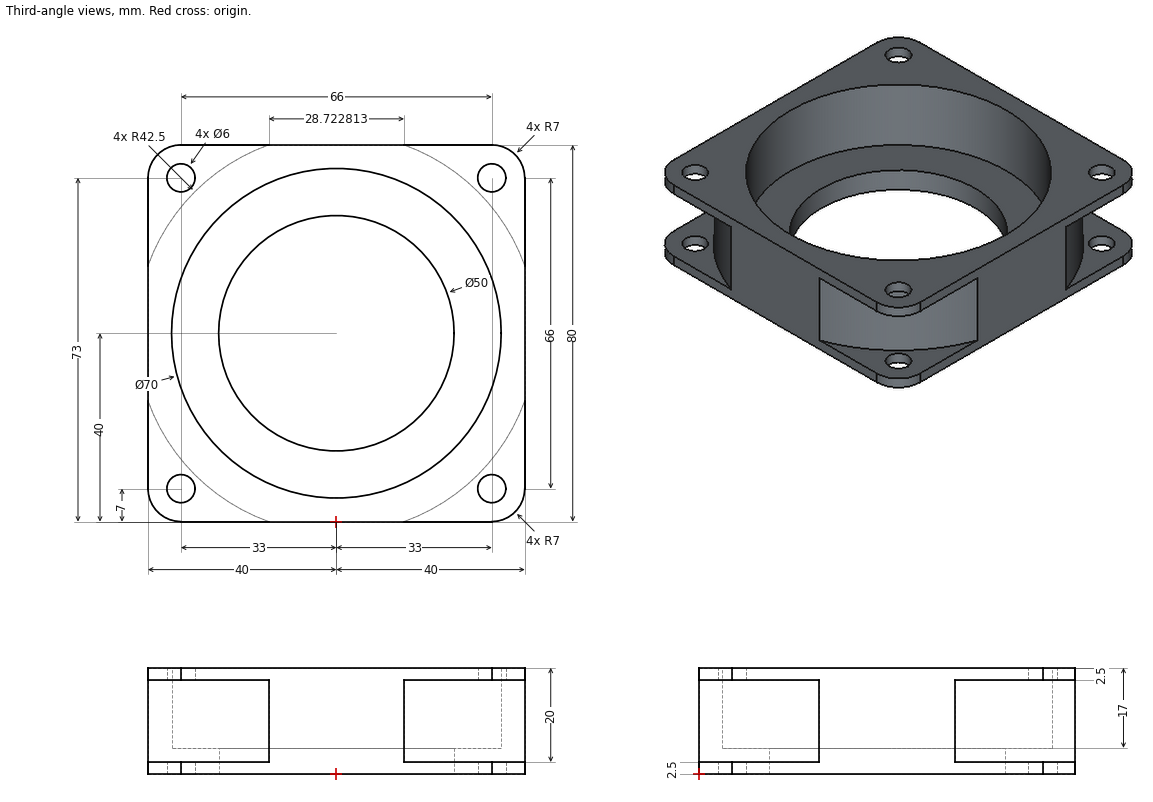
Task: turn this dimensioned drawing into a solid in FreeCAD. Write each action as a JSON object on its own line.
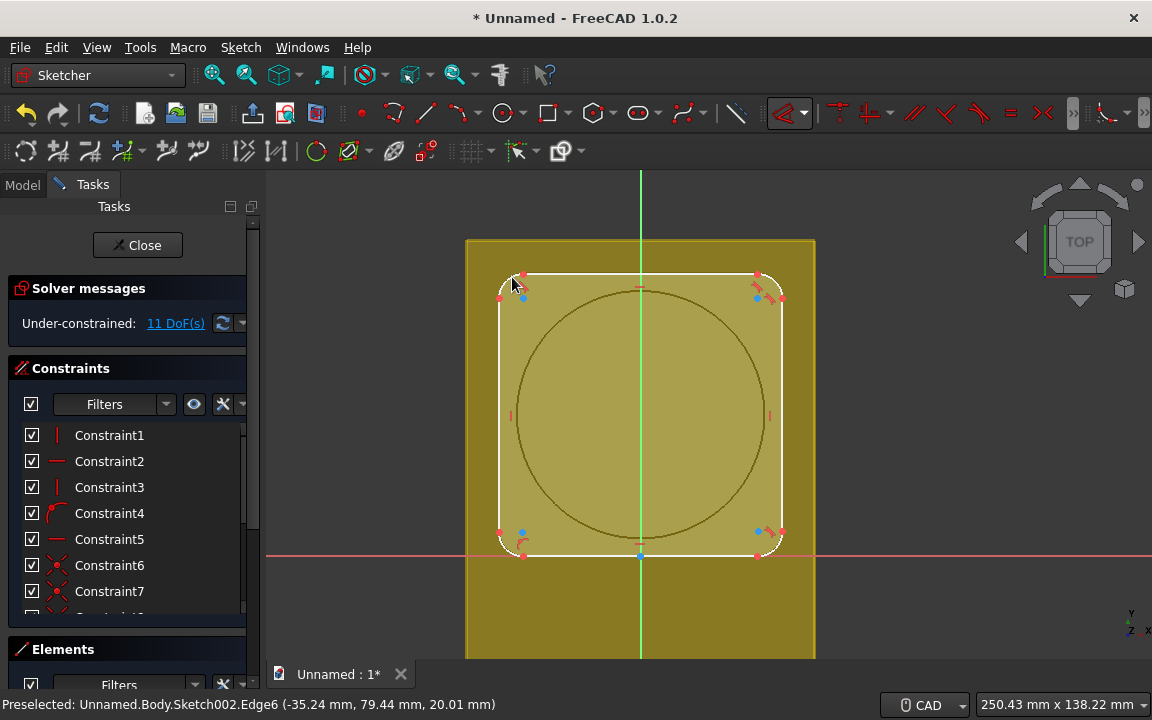
{"action": "left_click", "coordinate": [499, 369]}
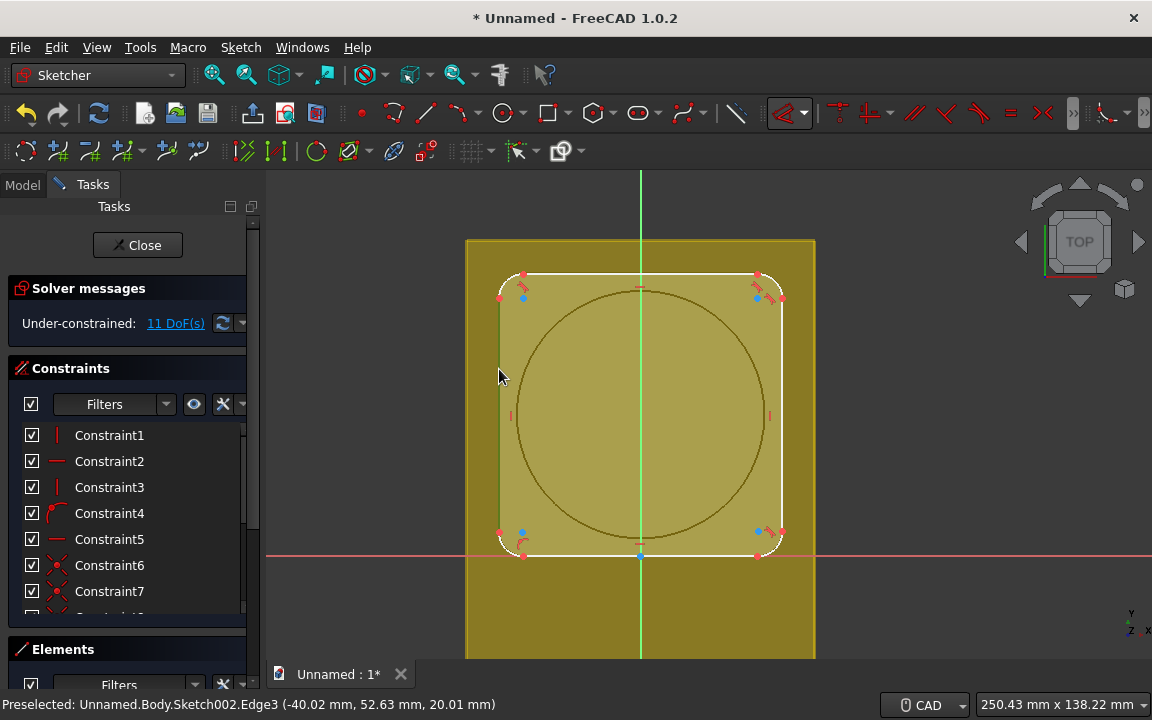
{"action": "left_click", "coordinate": [512, 277]}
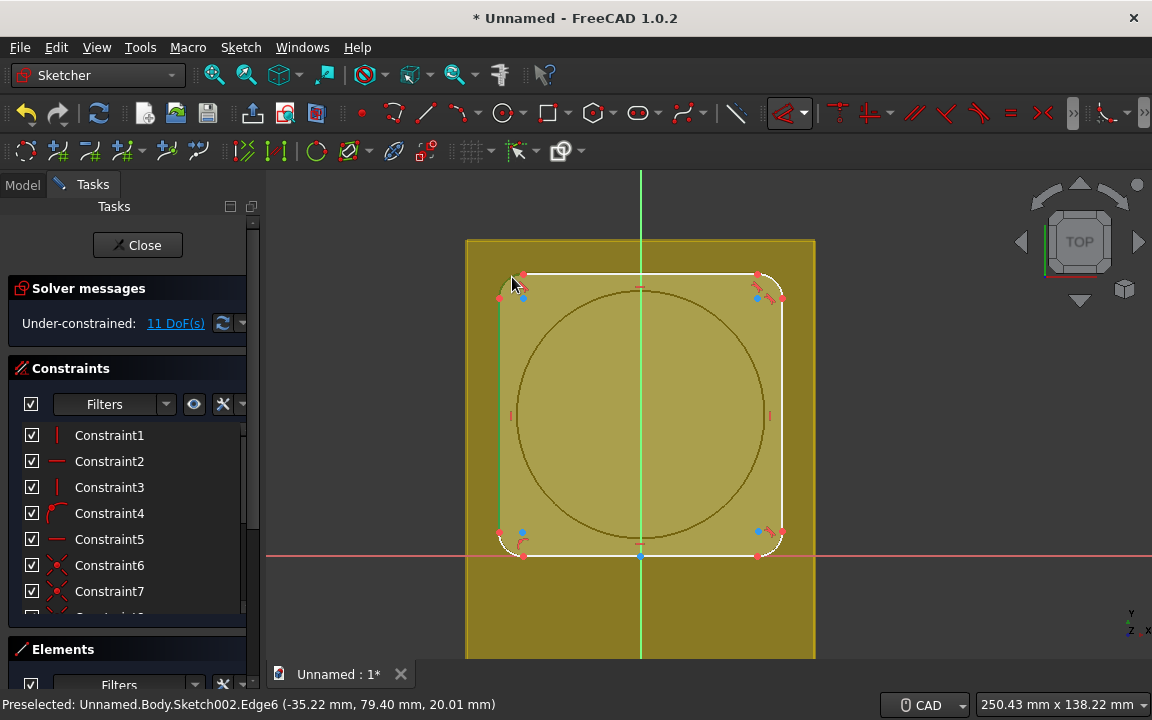
{"action": "left_click", "coordinate": [980, 114]}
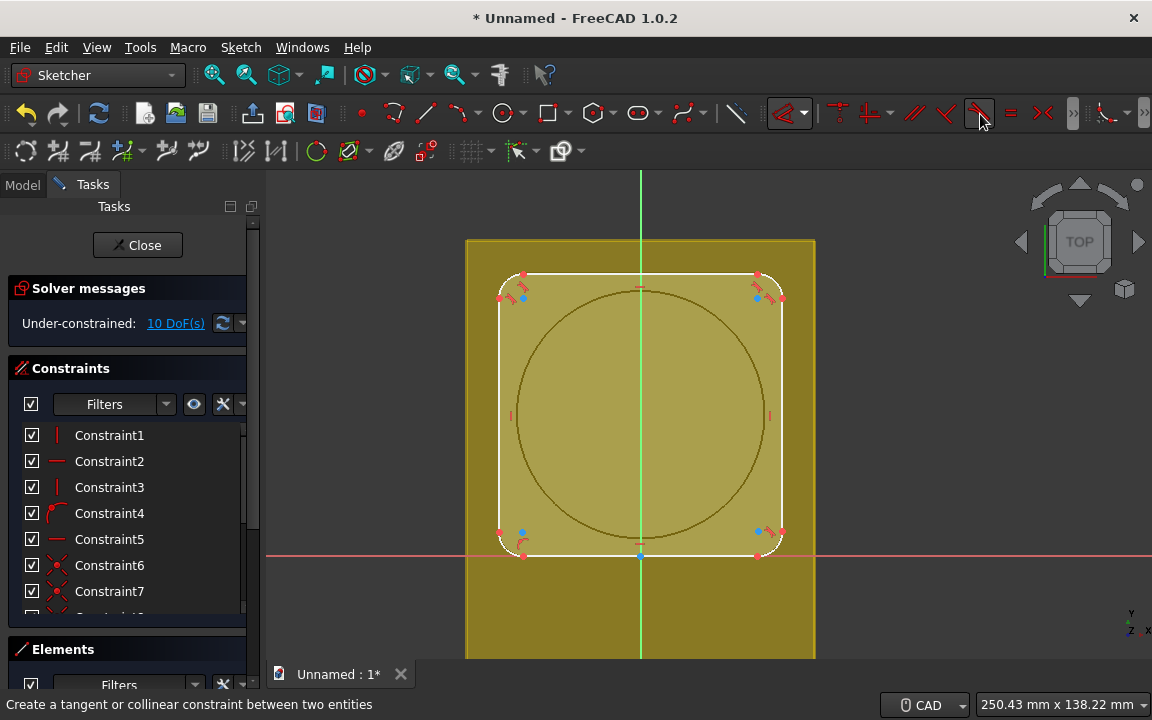
{"action": "left_click", "coordinate": [499, 369]}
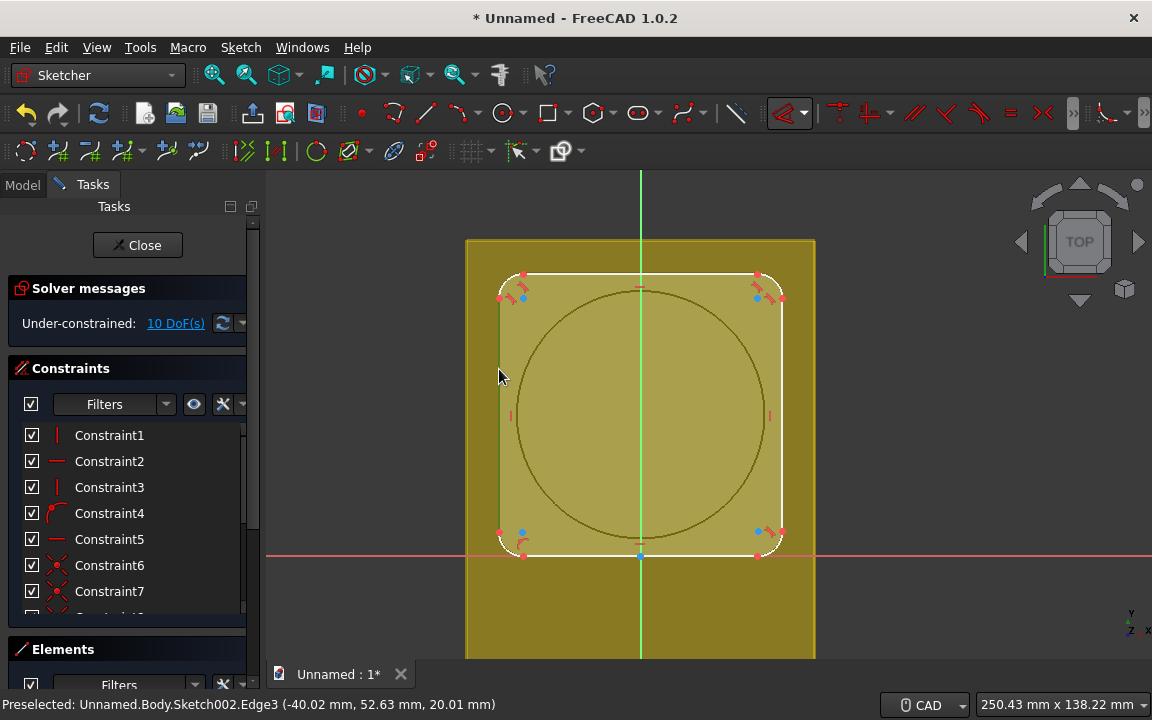
{"action": "left_click", "coordinate": [502, 543]}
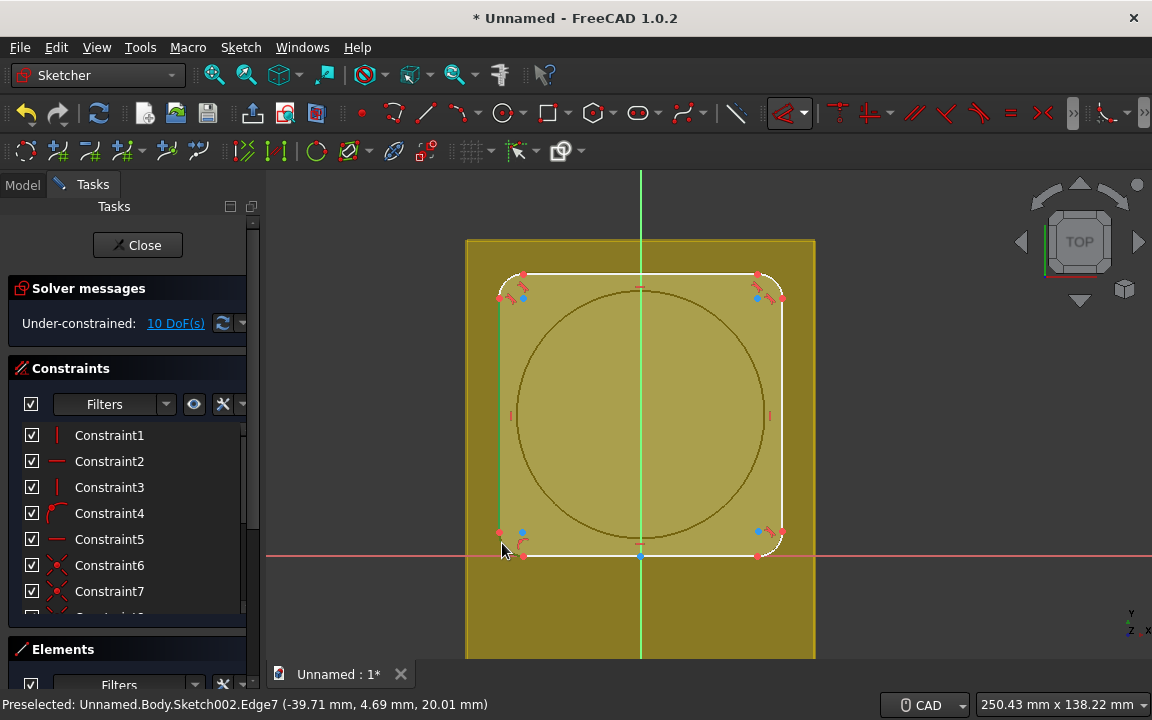
{"action": "left_click", "coordinate": [980, 114]}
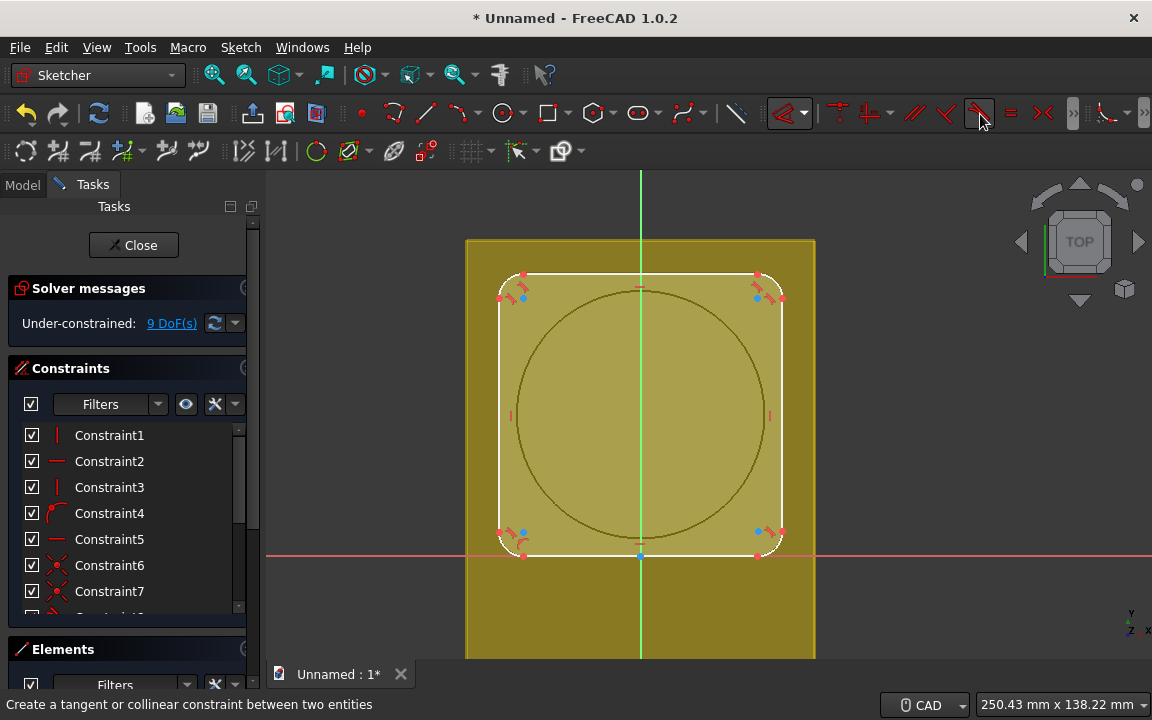
{"action": "left_click", "coordinate": [594, 556]}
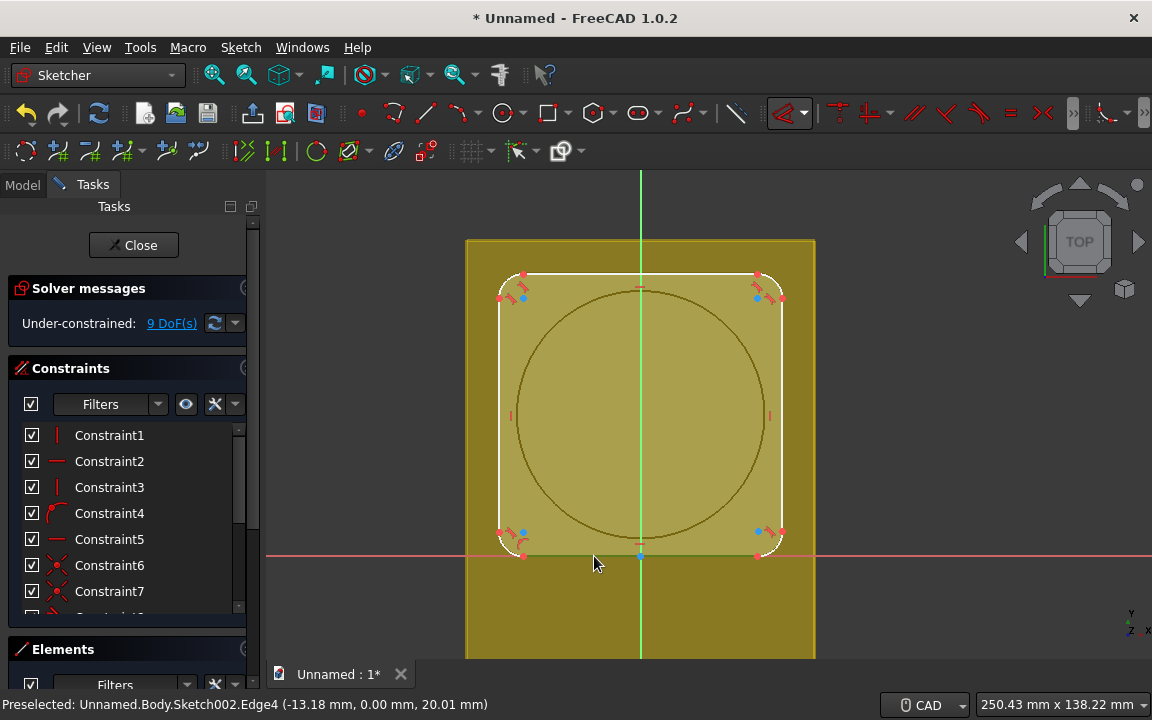
{"action": "left_click", "coordinate": [502, 543]}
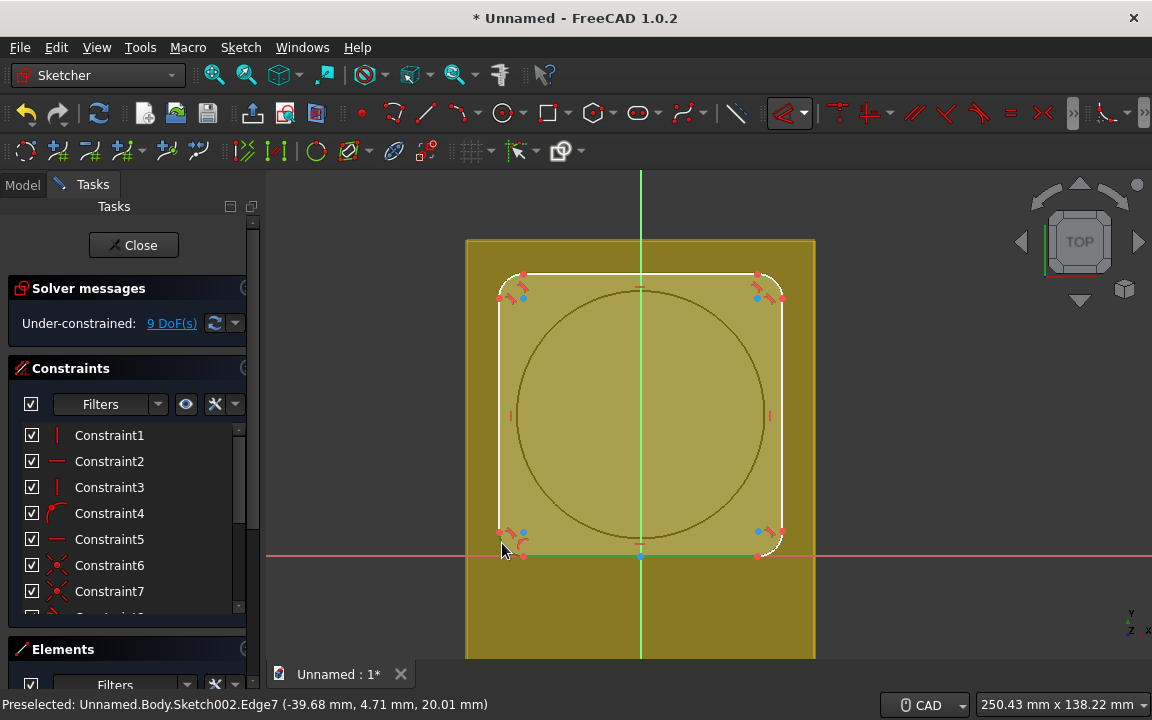
{"action": "key", "text": "t"}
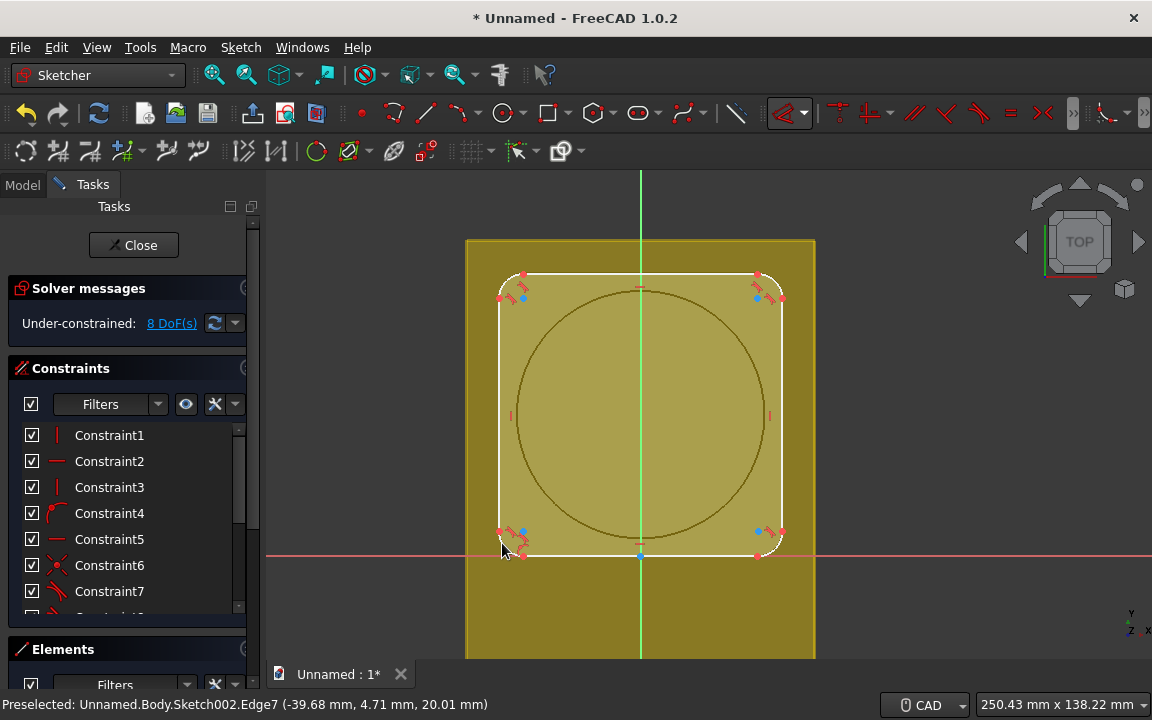
{"action": "left_click", "coordinate": [594, 556]}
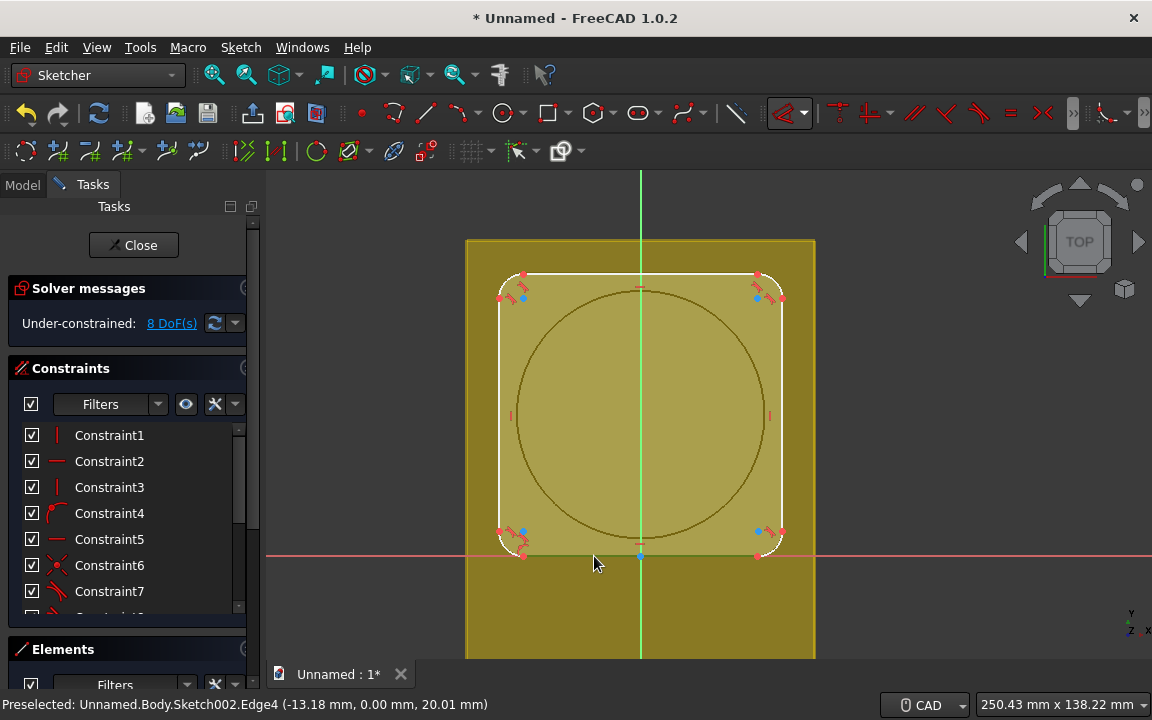
{"action": "left_click", "coordinate": [769, 554]}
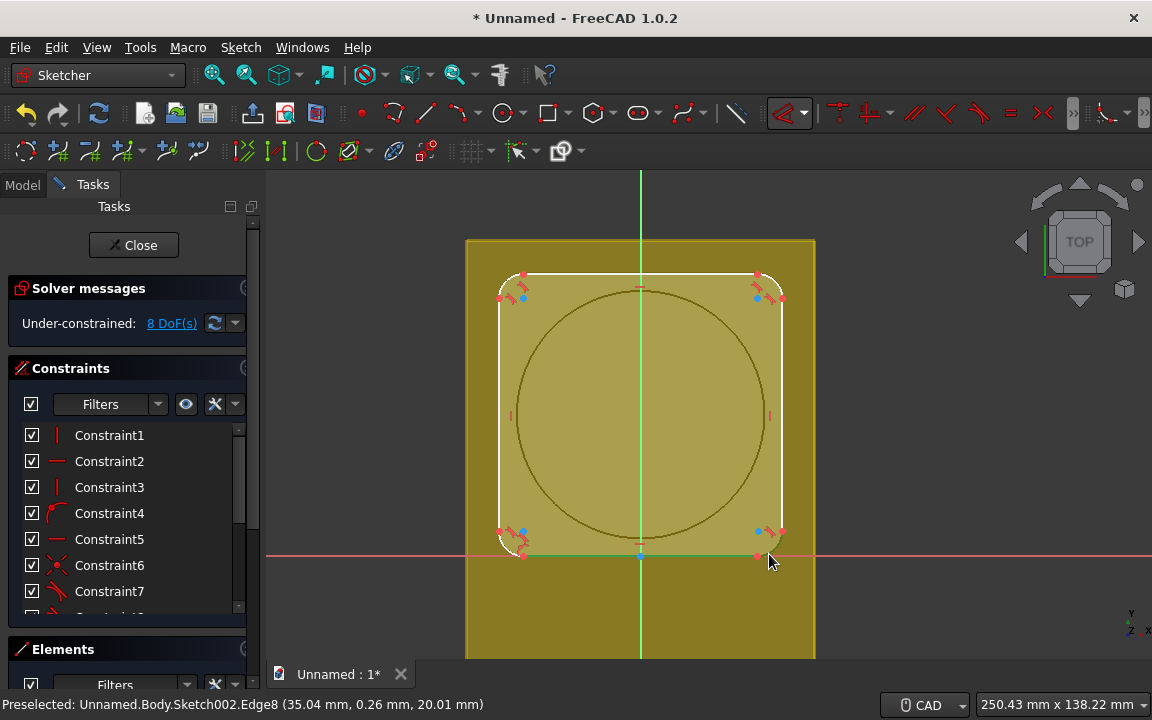
{"action": "key", "text": "t"}